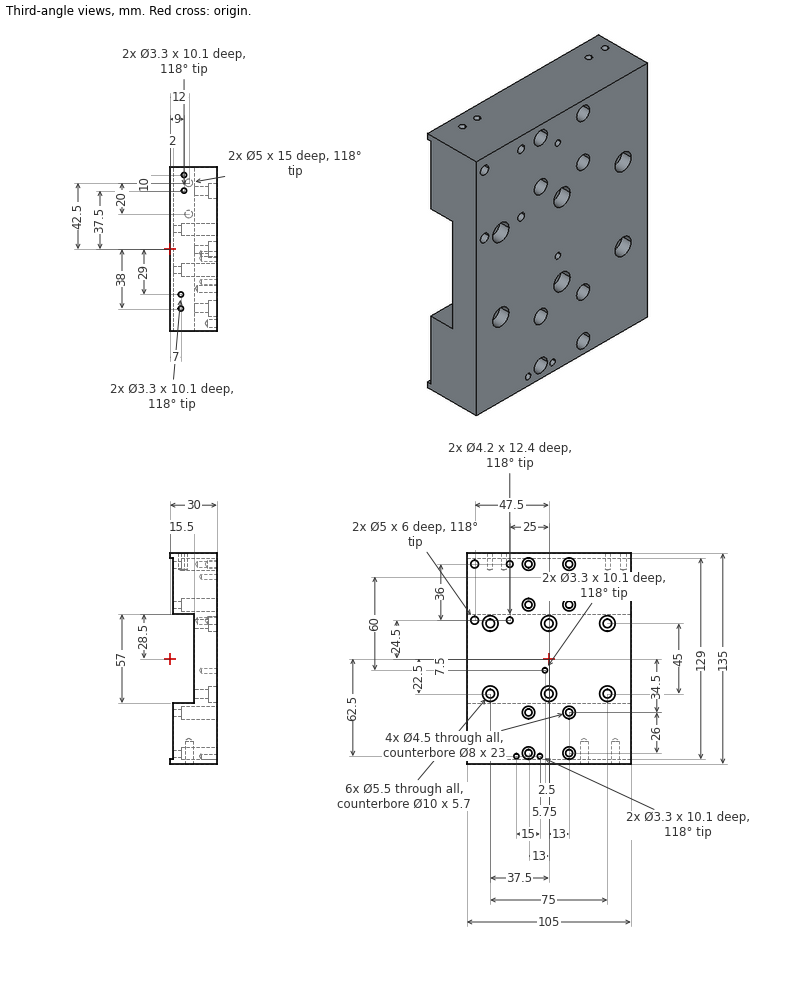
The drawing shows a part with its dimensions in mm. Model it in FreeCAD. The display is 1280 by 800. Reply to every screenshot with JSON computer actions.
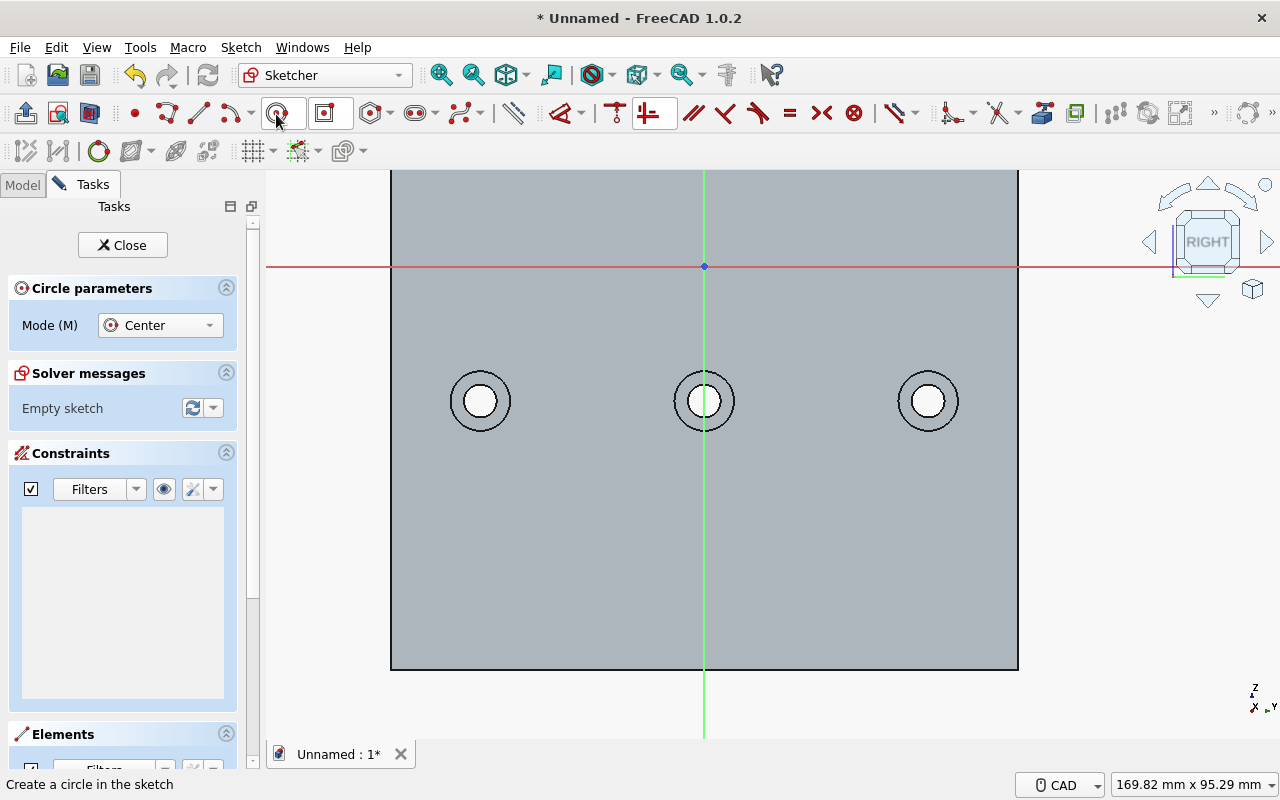
{"action": "scroll", "coordinate": [782, 473], "scroll_direction": "up", "scroll_amount": 3}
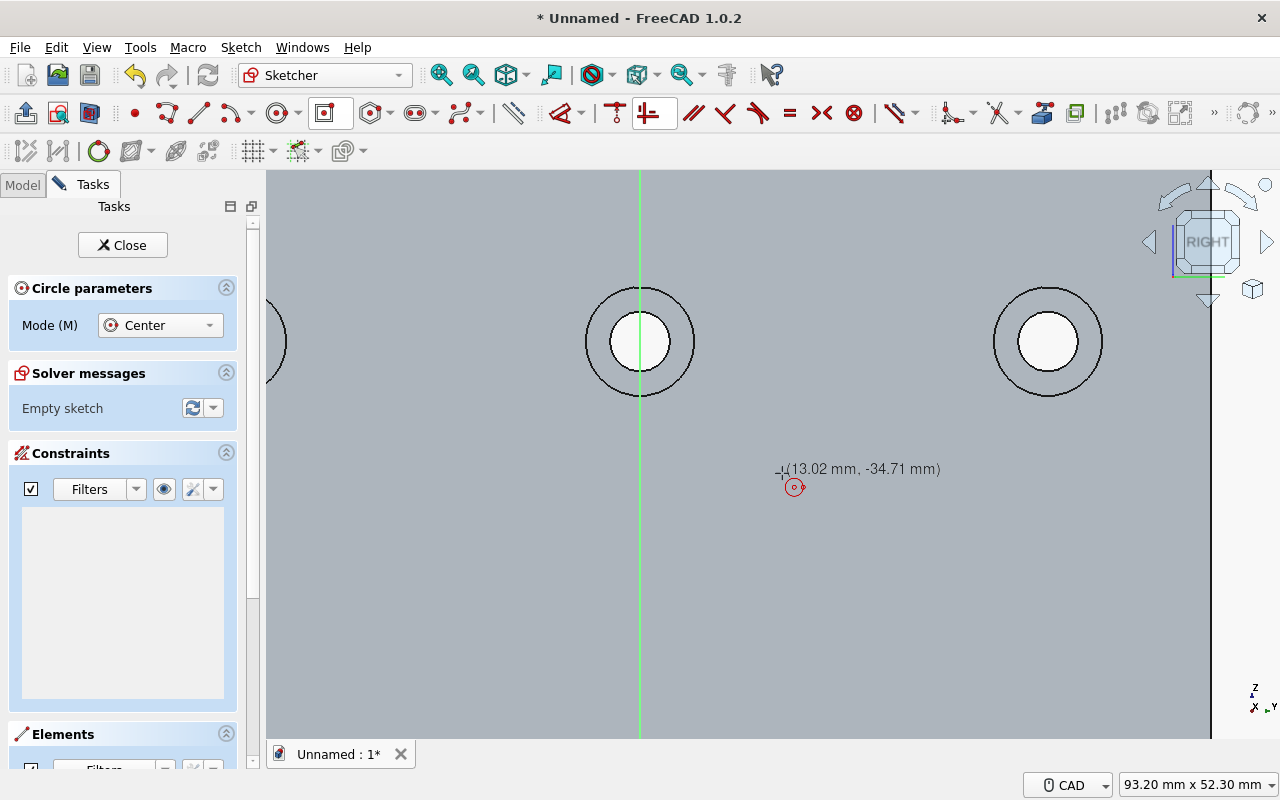
{"action": "left_click", "coordinate": [781, 472]}
{"action": "left_click", "coordinate": [799, 455]}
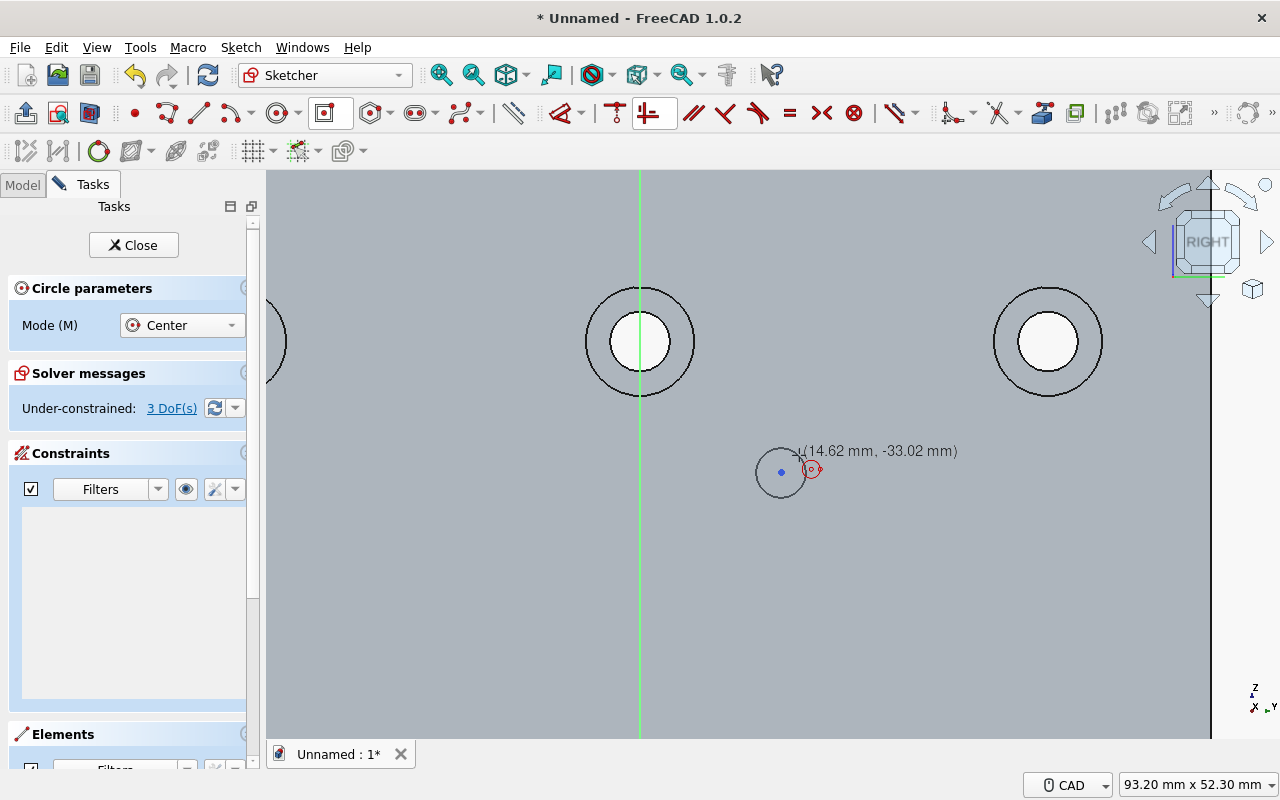
{"action": "scroll", "coordinate": [783, 474], "scroll_direction": "down", "scroll_amount": 3}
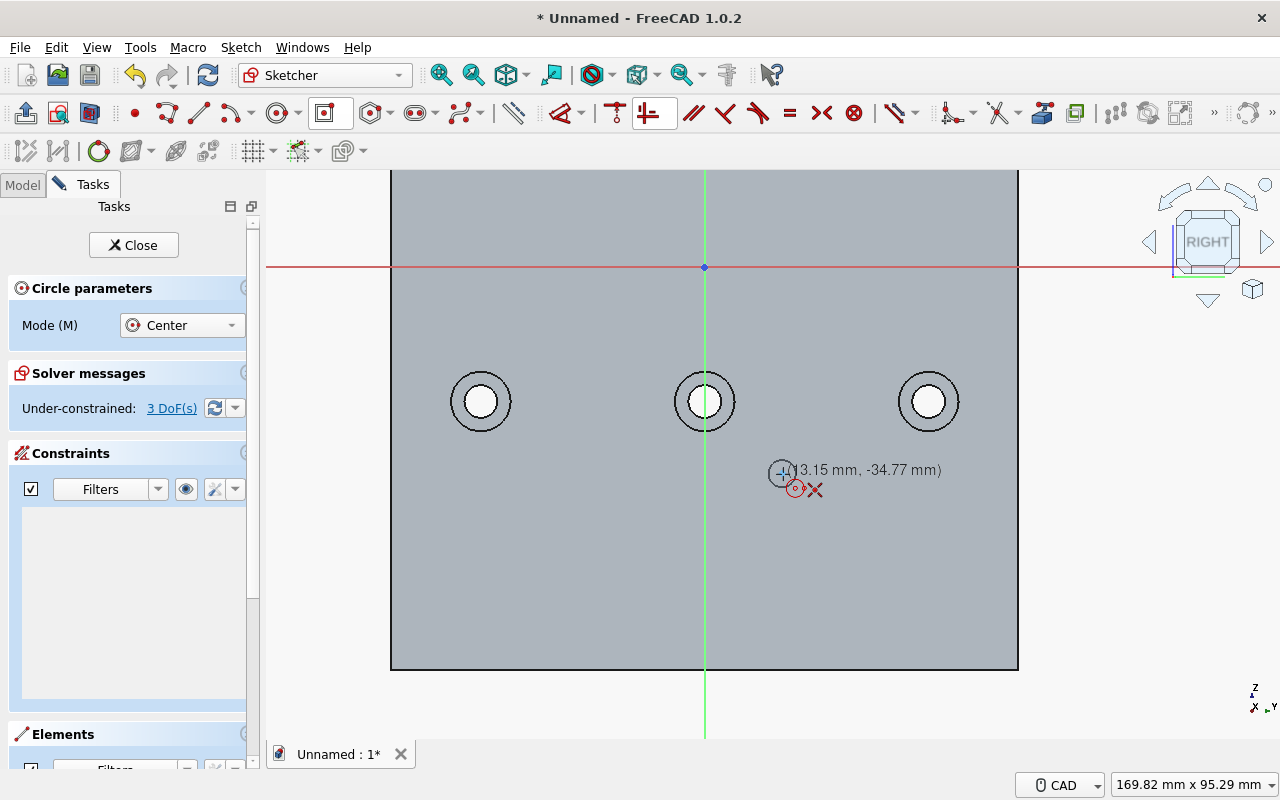
{"action": "scroll", "coordinate": [782, 628], "scroll_direction": "up", "scroll_amount": 3}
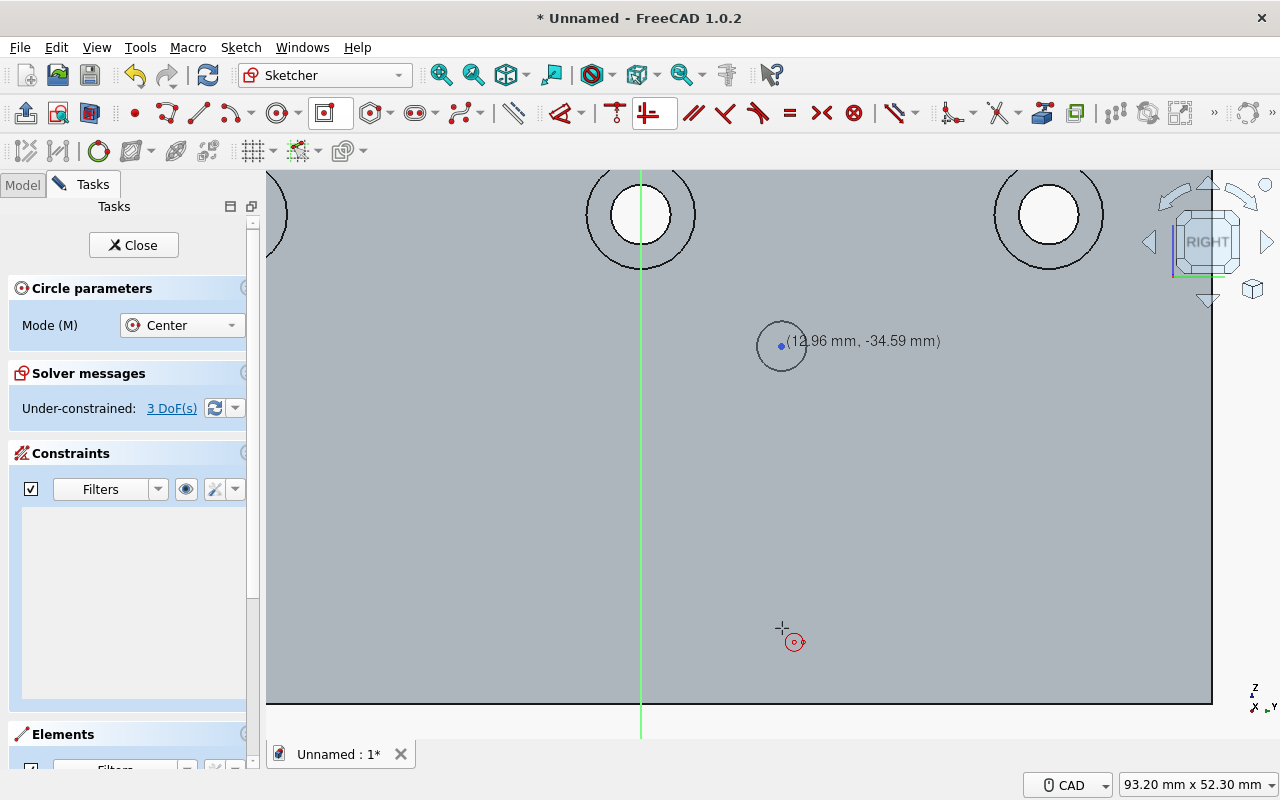
{"action": "left_click", "coordinate": [782, 628]}
{"action": "left_click", "coordinate": [800, 611]}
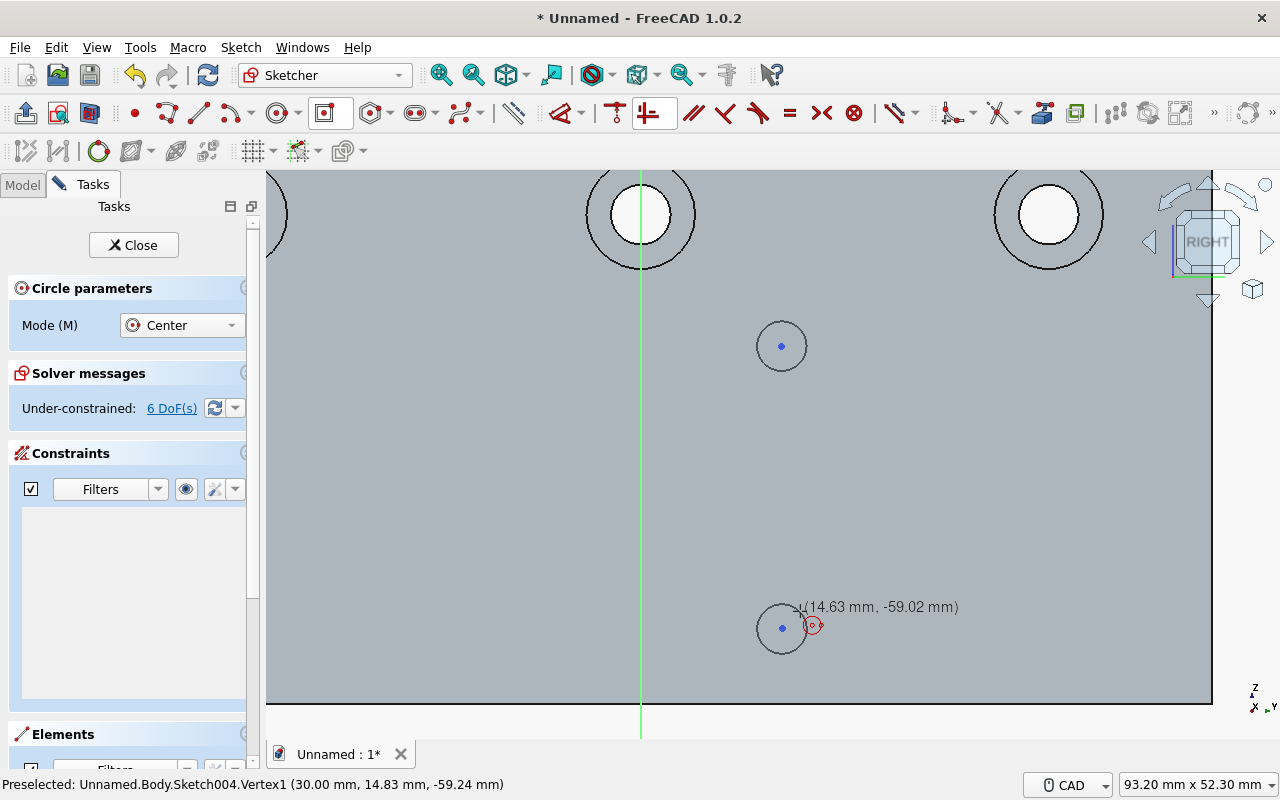
{"action": "left_click", "coordinate": [499, 628]}
{"action": "left_click", "coordinate": [517, 611]}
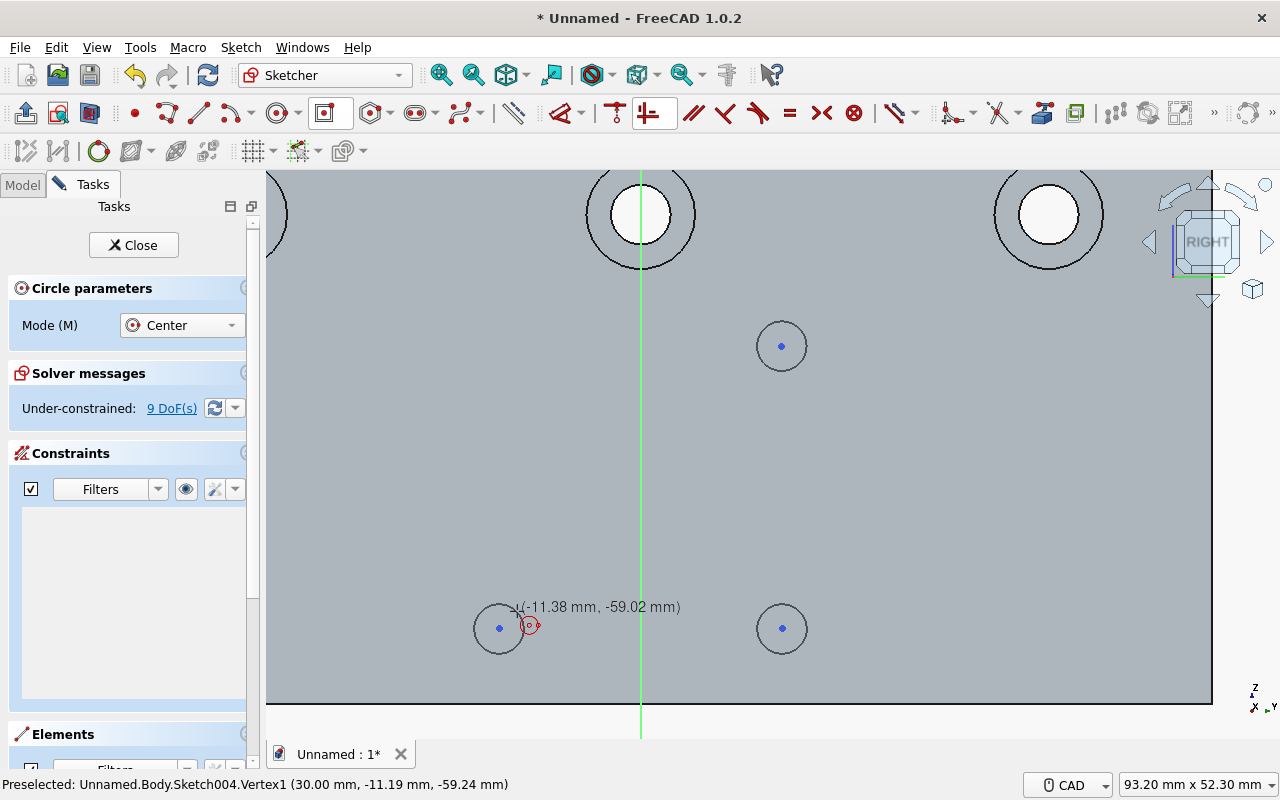
{"action": "left_click", "coordinate": [499, 345]}
{"action": "left_click", "coordinate": [517, 328]}
{"action": "key", "text": "Escape"}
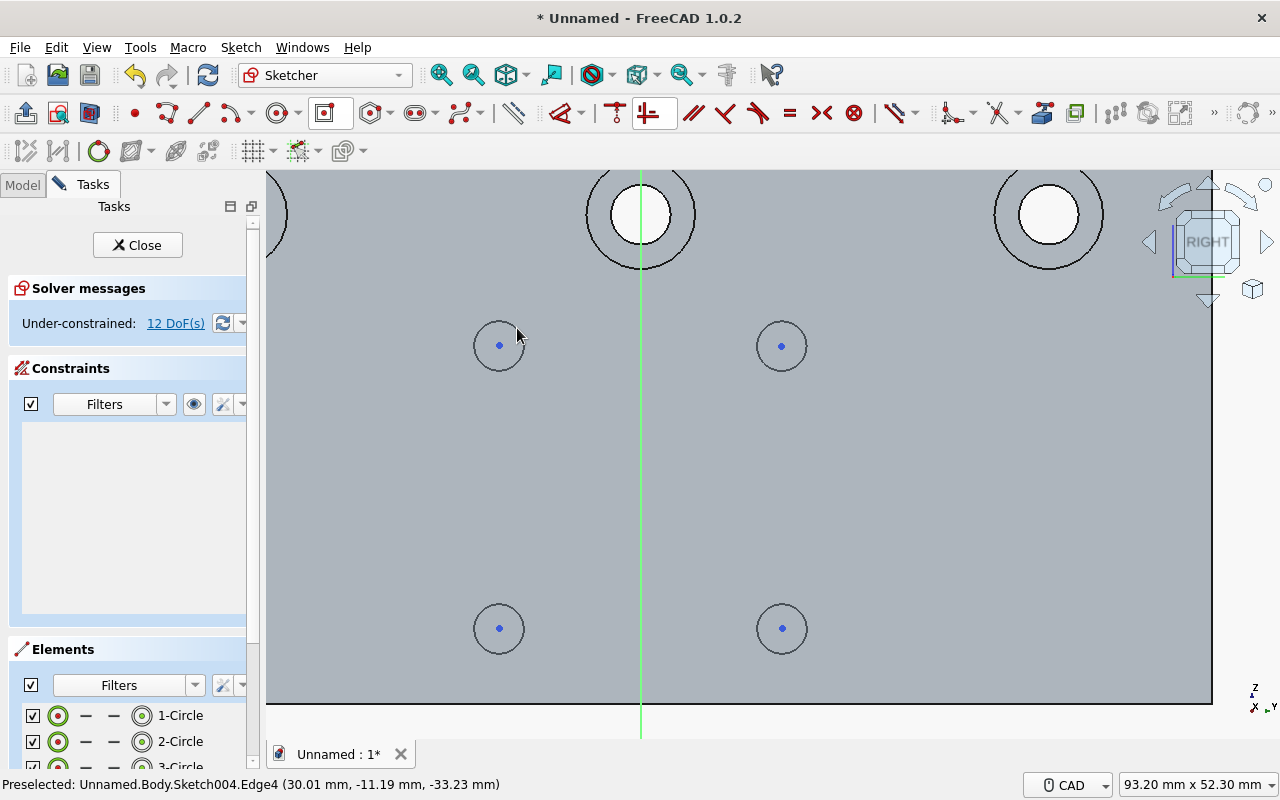
{"action": "left_click", "coordinate": [799, 329]}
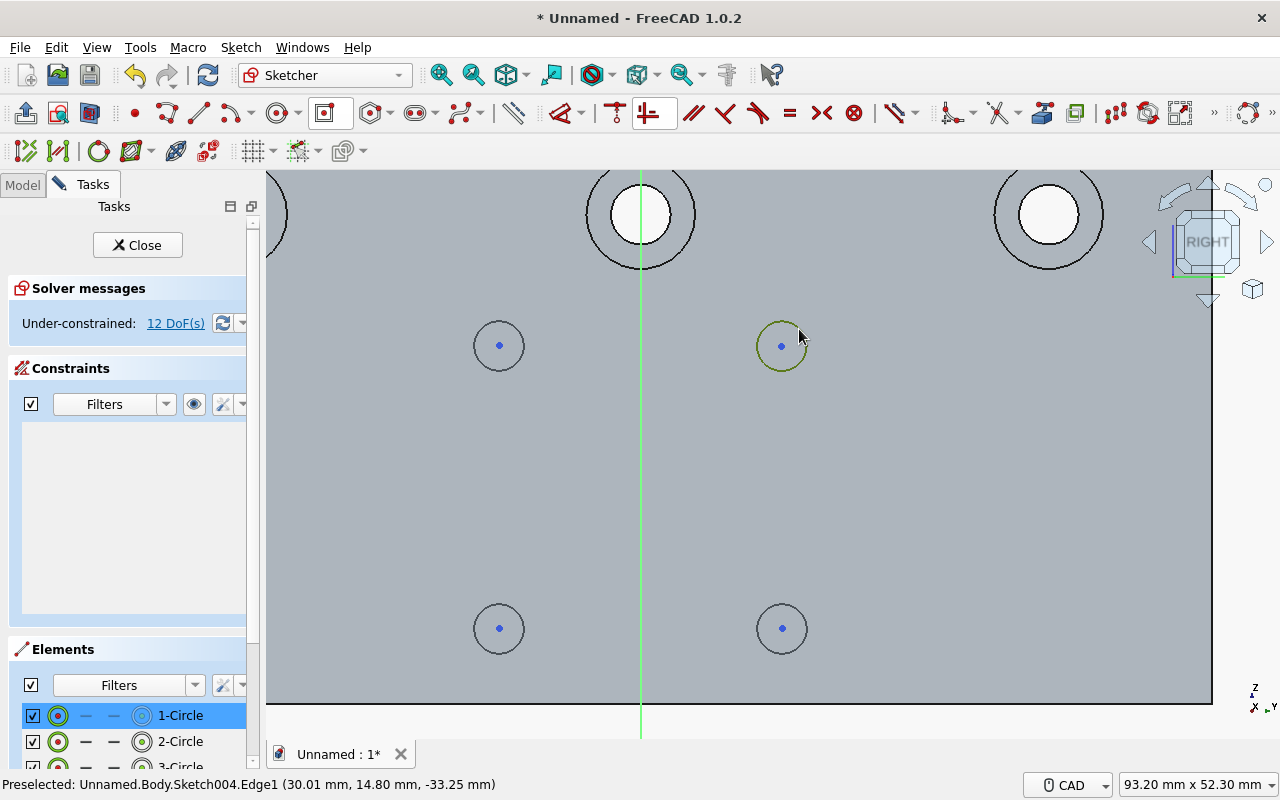
{"action": "left_click", "coordinate": [799, 611]}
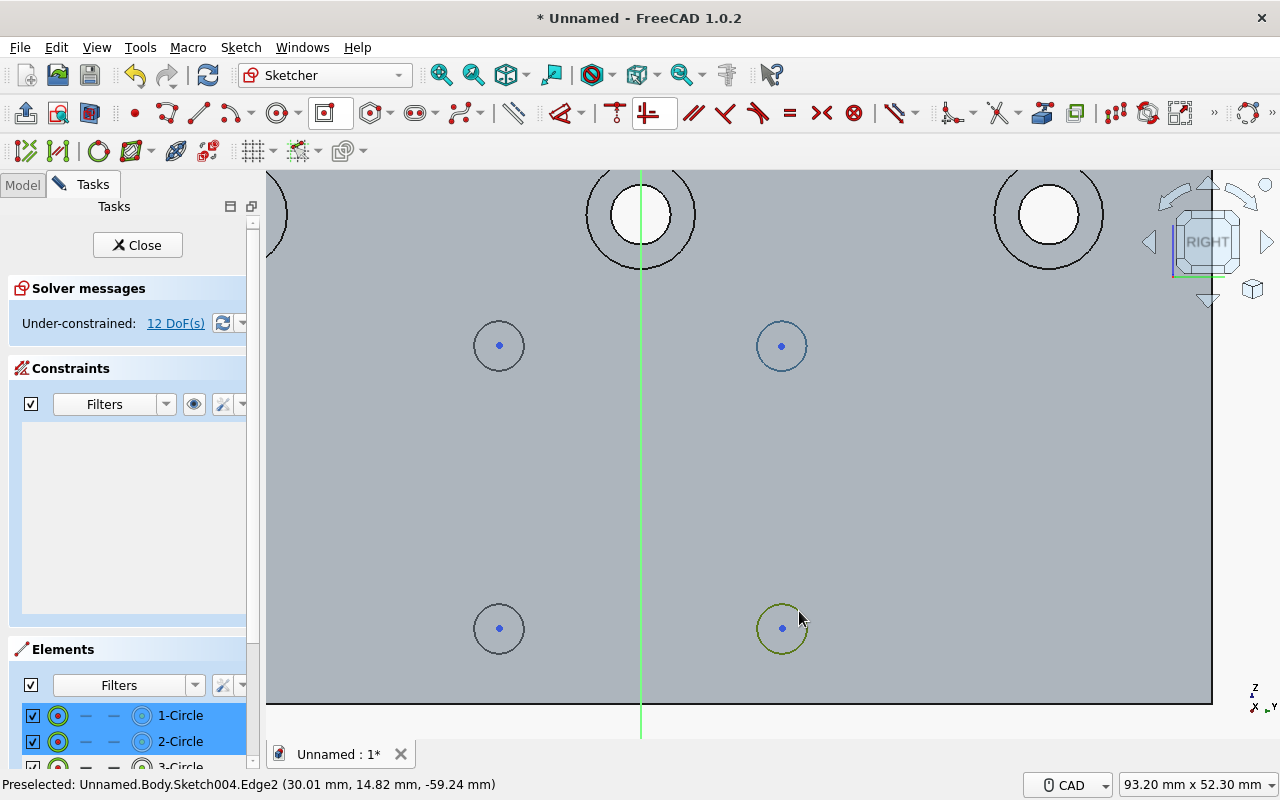
{"action": "left_click", "coordinate": [516, 611]}